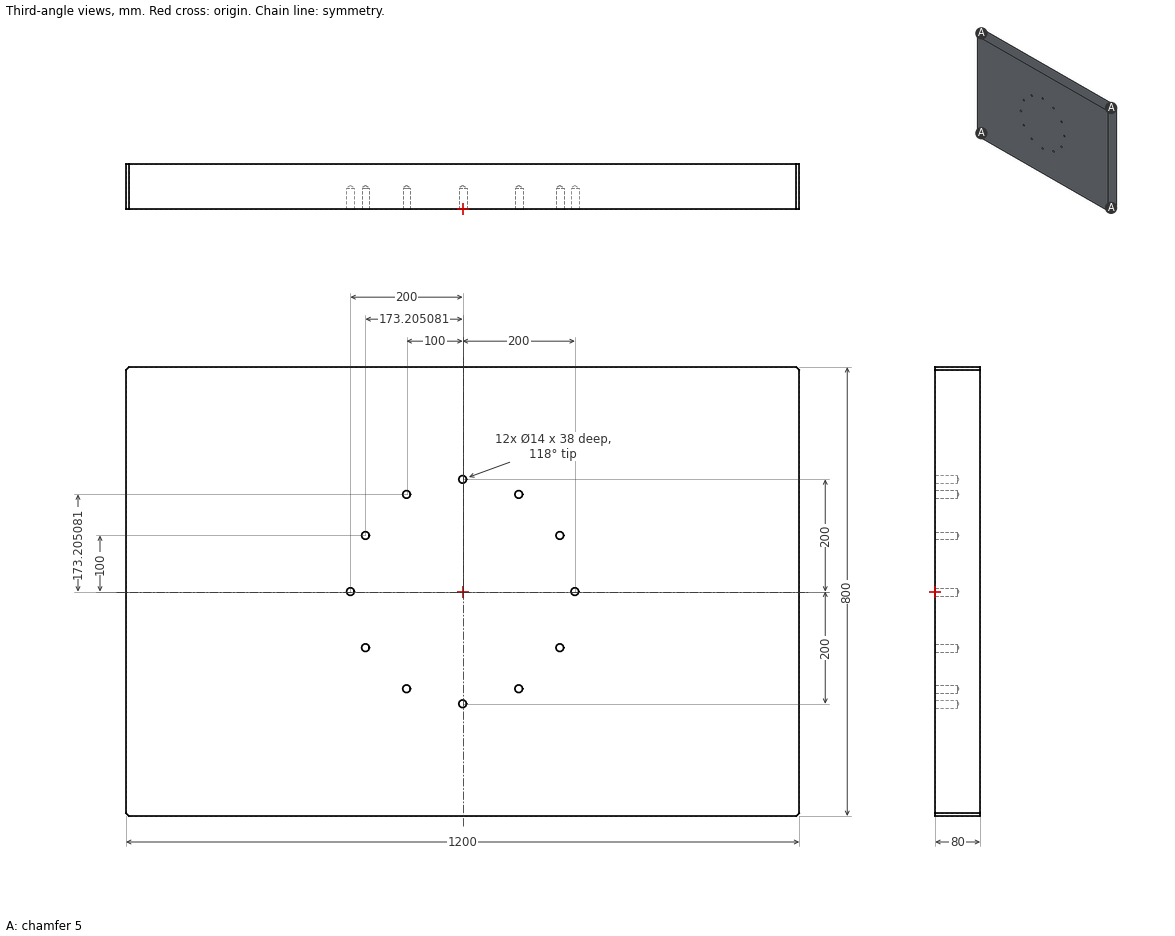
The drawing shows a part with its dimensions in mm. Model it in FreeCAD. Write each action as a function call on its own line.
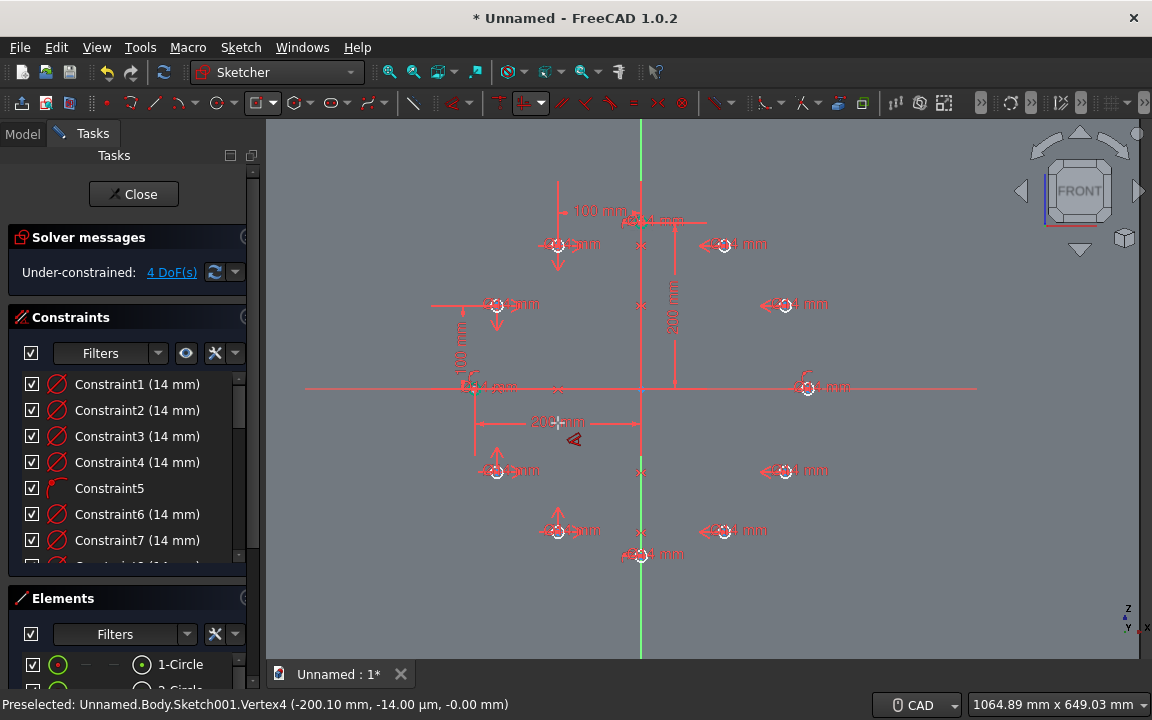
click(641, 556)
click(675, 473)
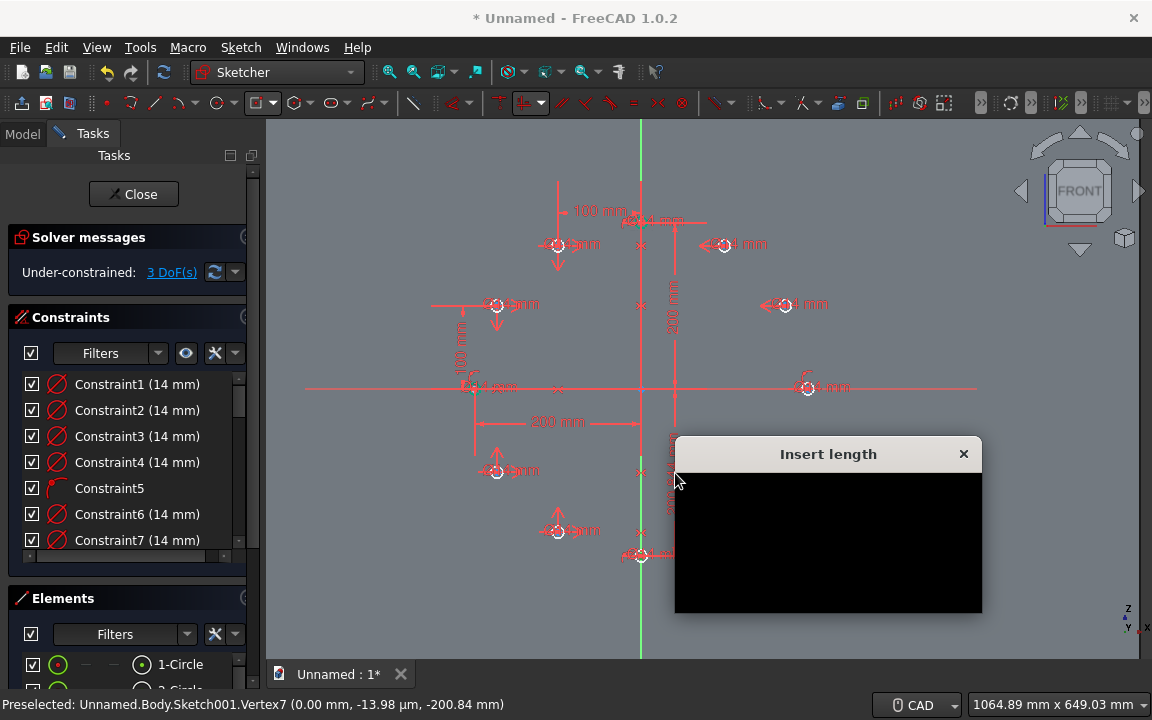
text(200)
key(Return)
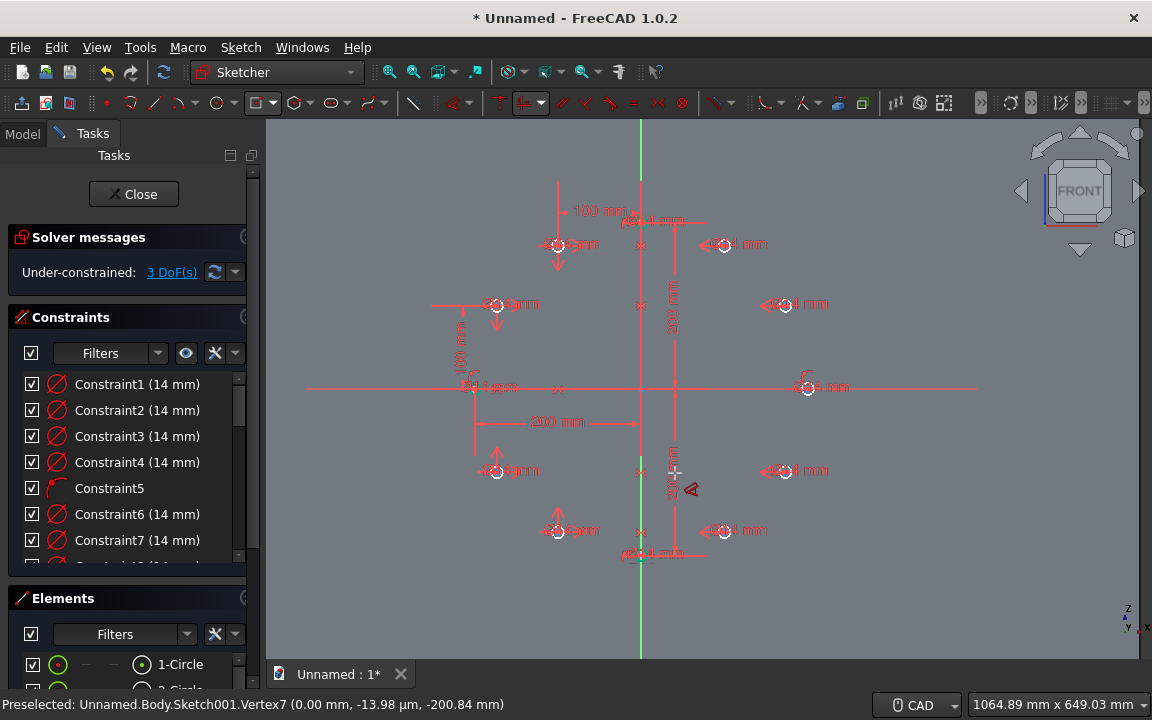
click(808, 389)
click(725, 423)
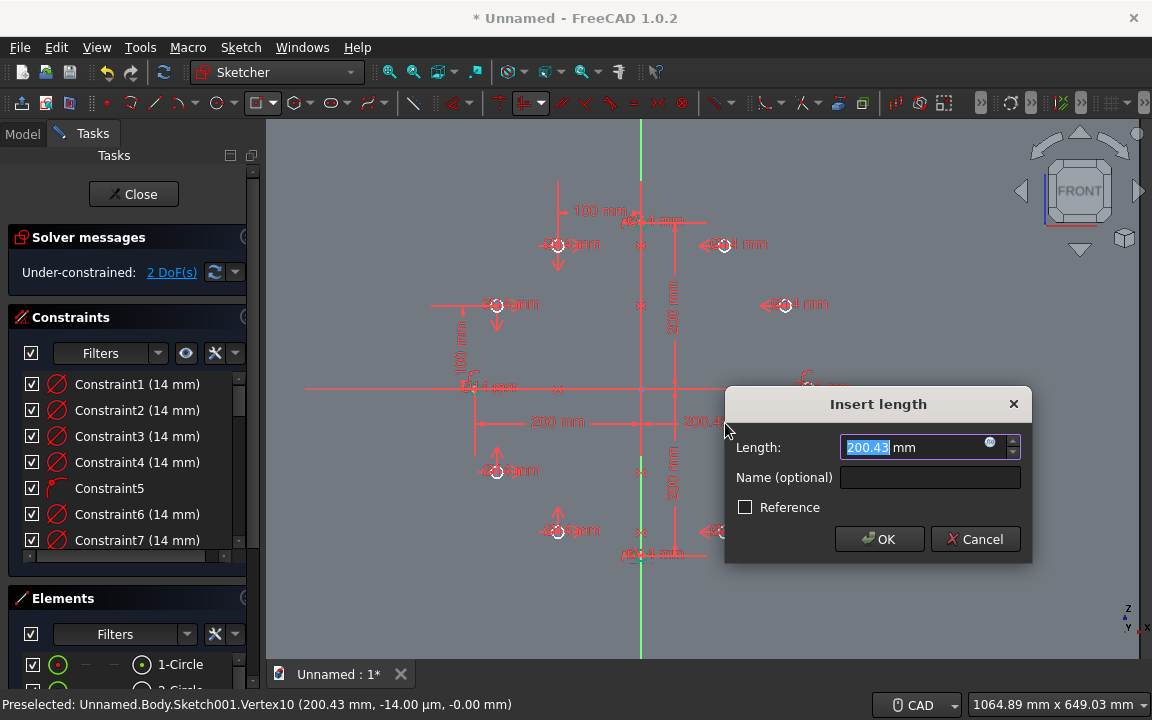
text(200)
key(Return)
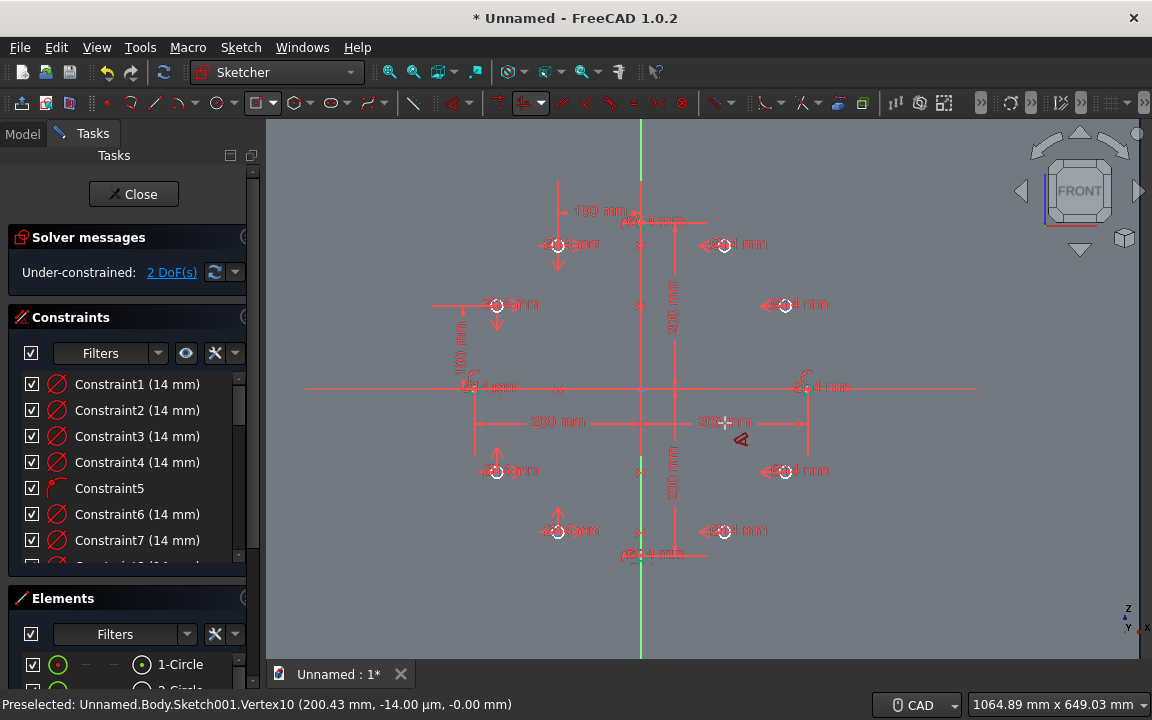
click(558, 246)
click(524, 318)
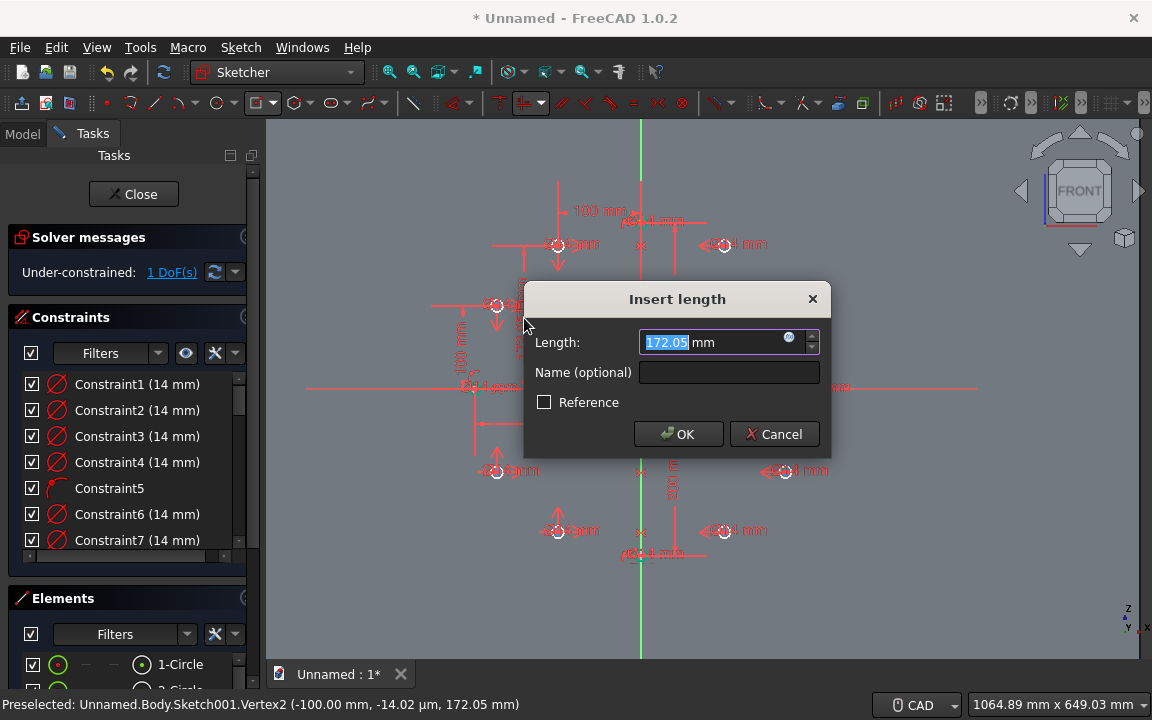
text(173.205081)
key(Return)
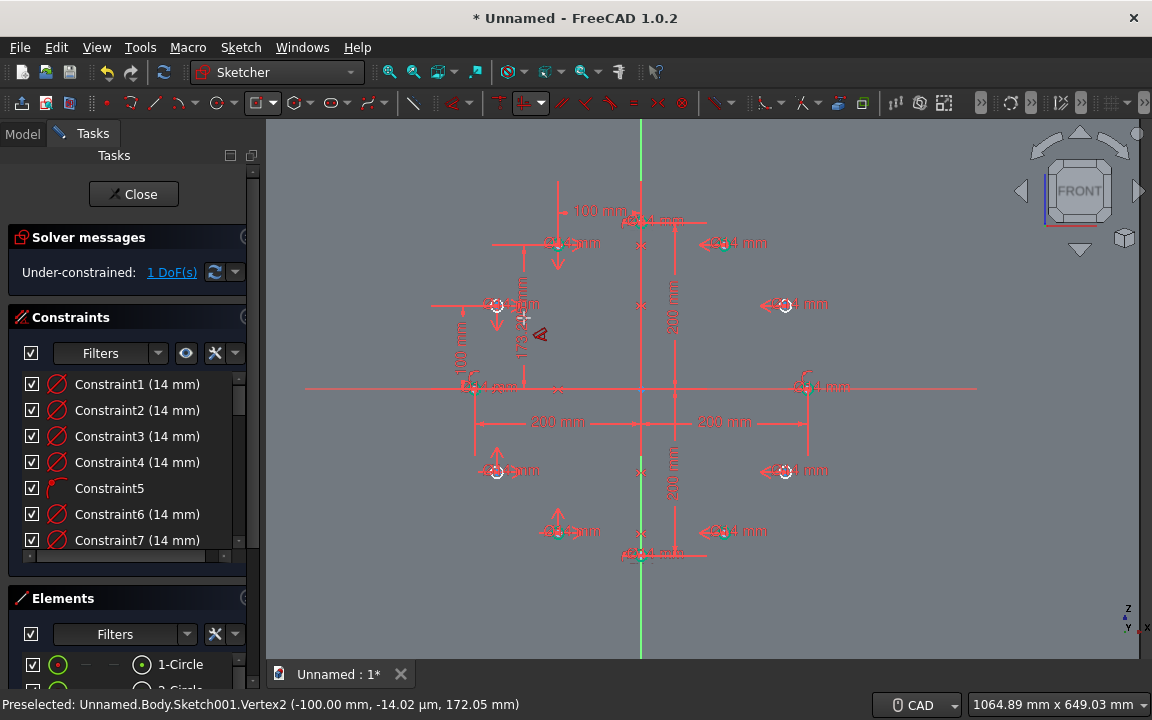
click(497, 306)
click(569, 272)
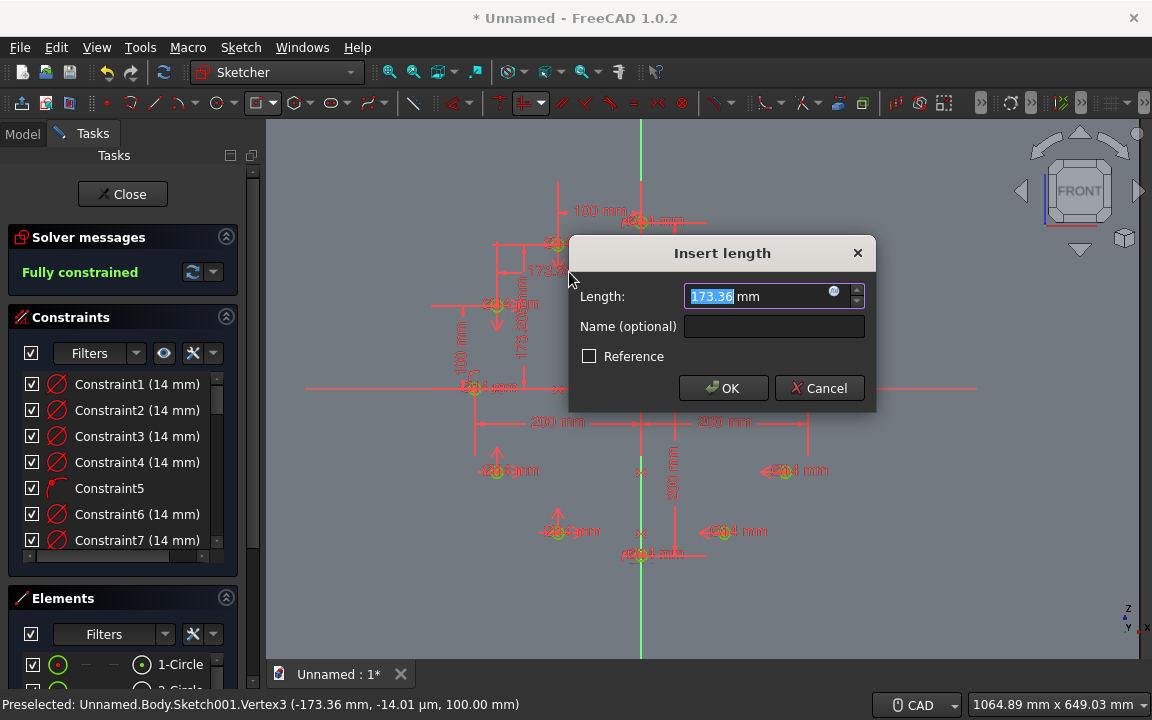
text(173.205081)
key(Return)
key(Escape)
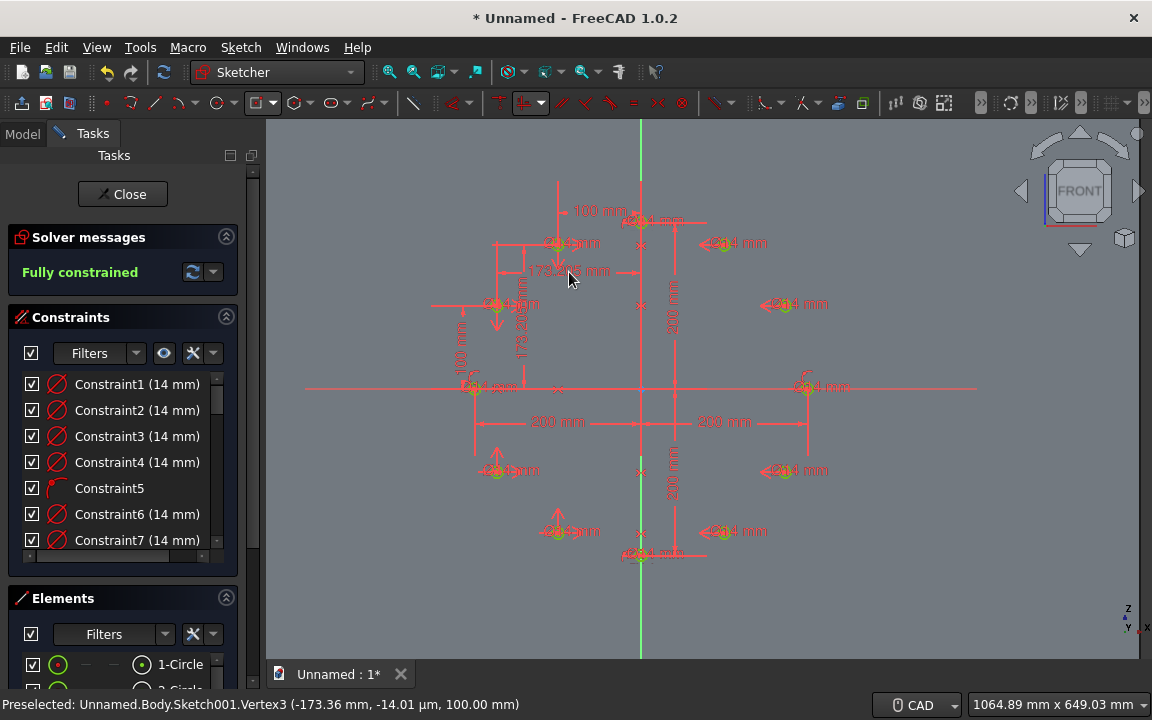
click(123, 194)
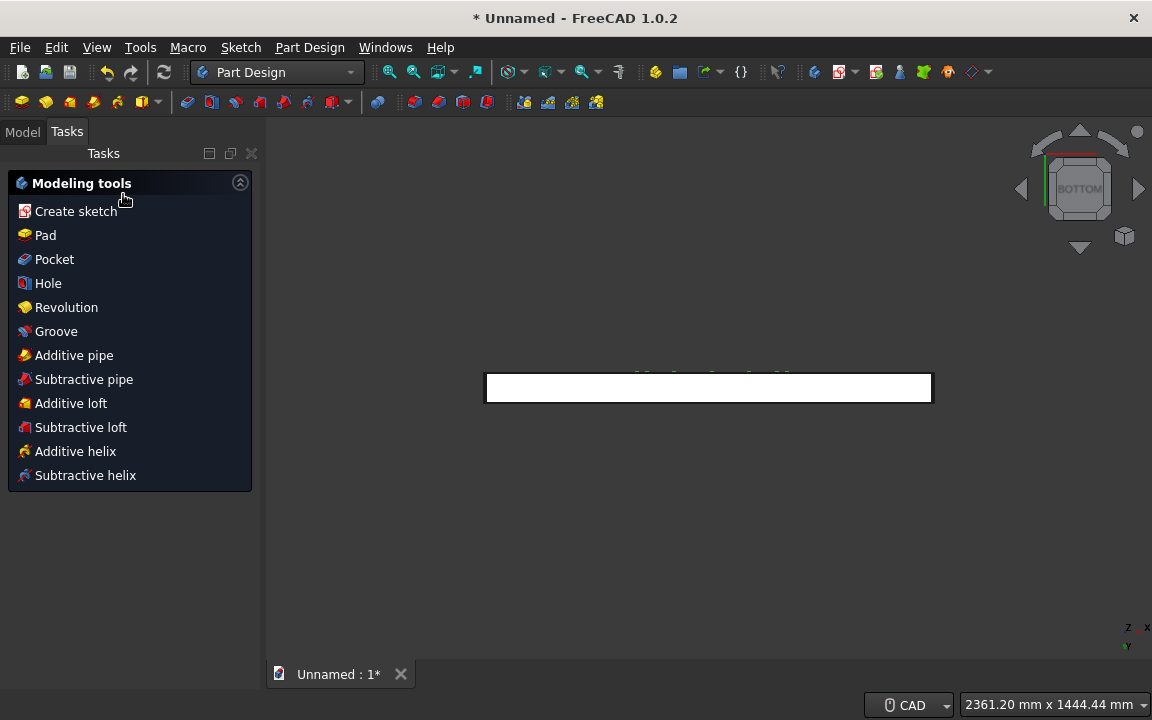
click(212, 102)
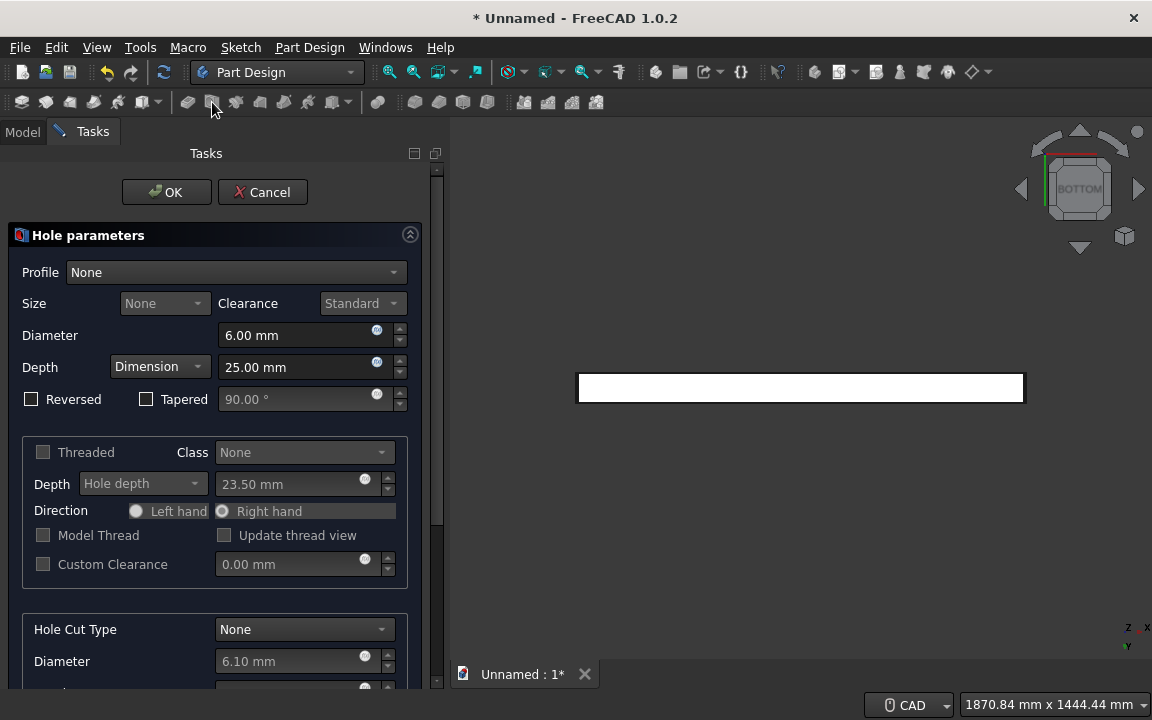
triple_click(305, 335)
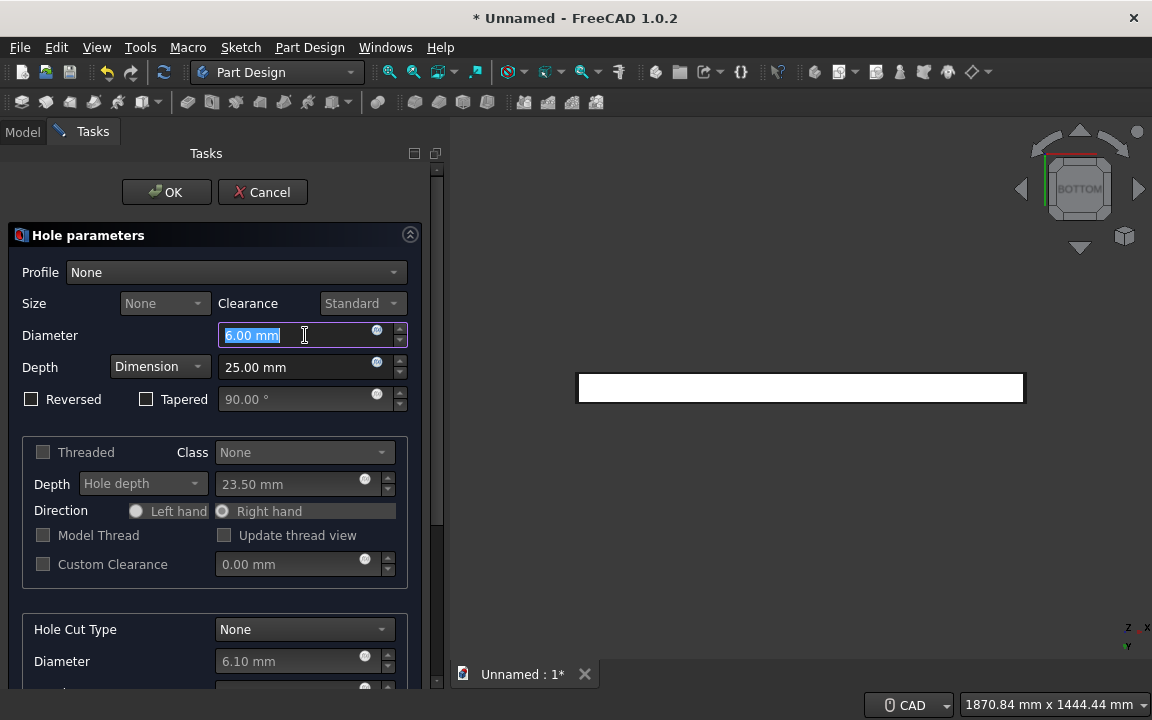
text(14)
key(Tab)